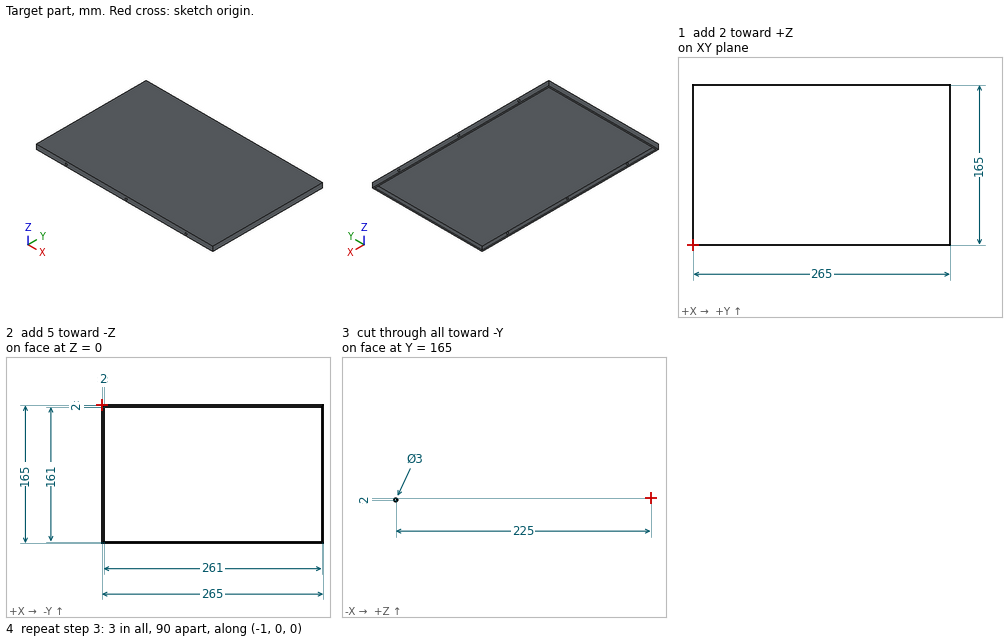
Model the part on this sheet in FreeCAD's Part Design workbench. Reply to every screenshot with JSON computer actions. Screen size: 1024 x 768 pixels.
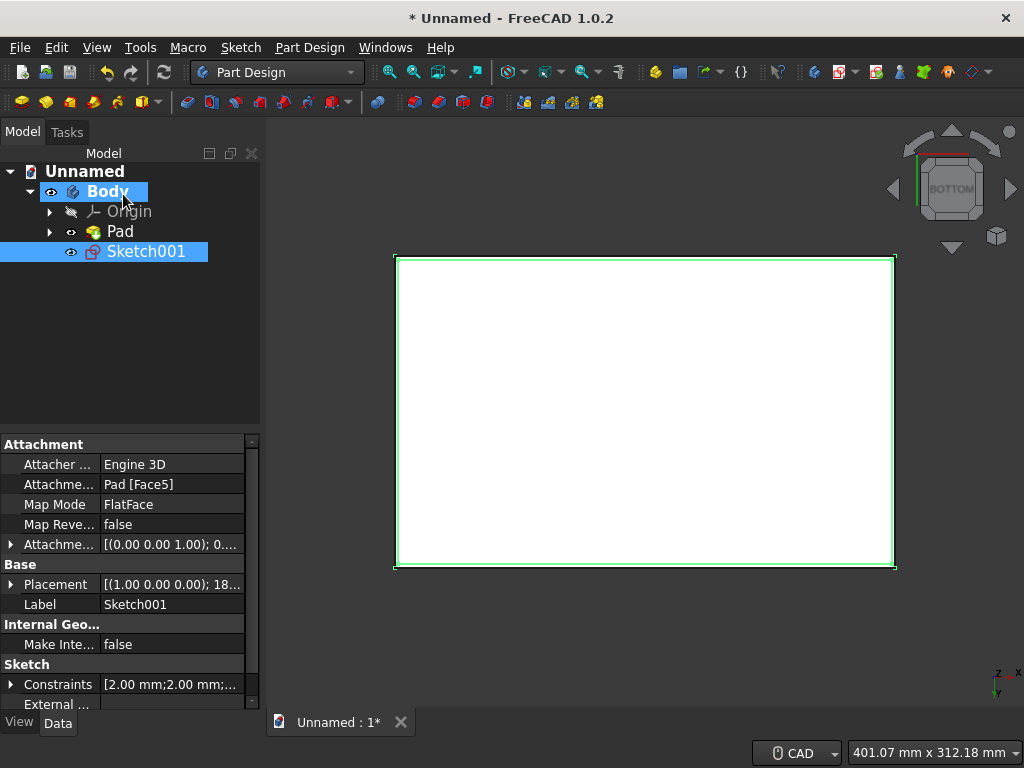
{"action": "left_click", "coordinate": [22, 102]}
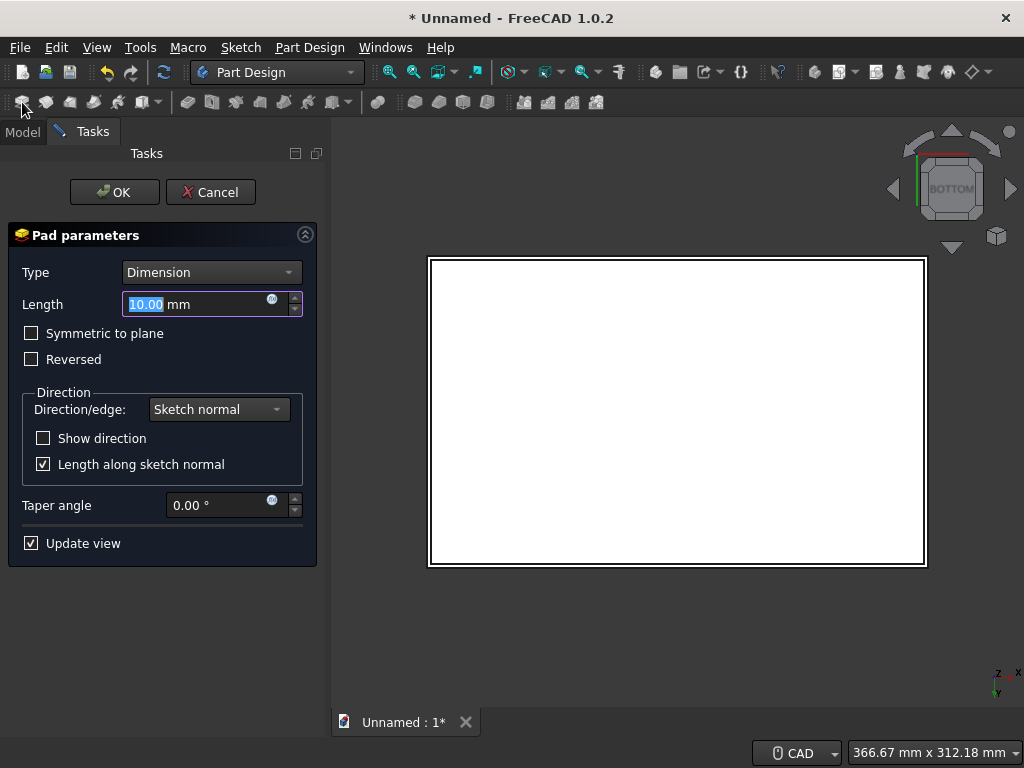
{"action": "type", "text": "5"}
{"action": "key", "text": "Tab"}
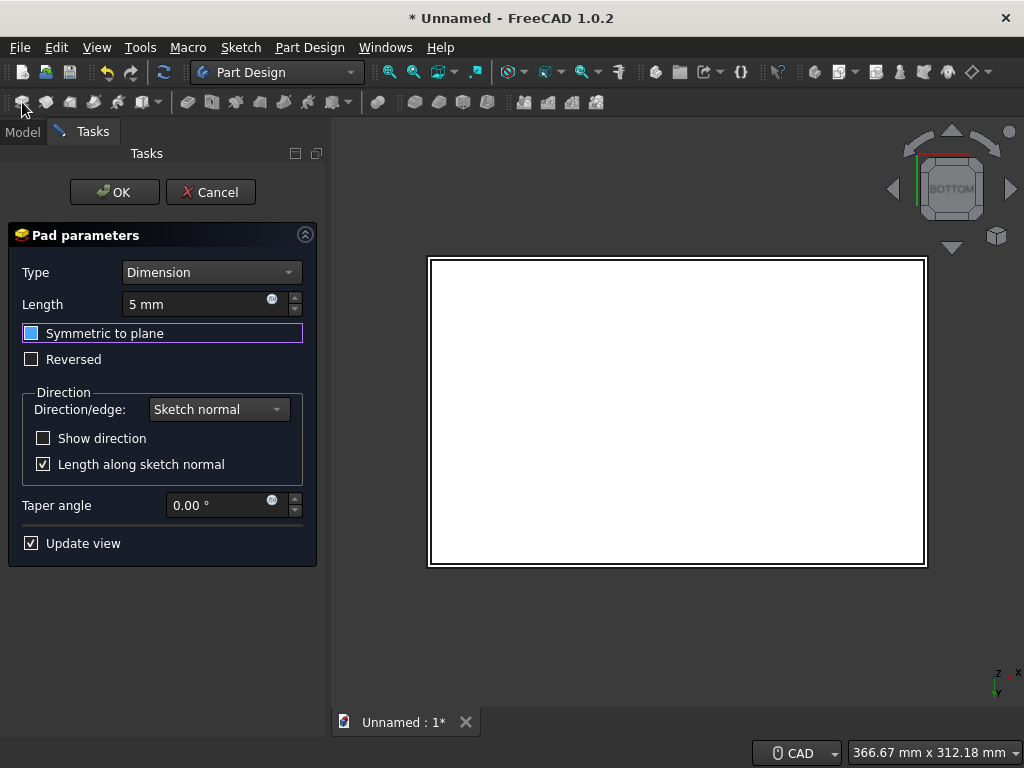
{"action": "left_click", "coordinate": [115, 192]}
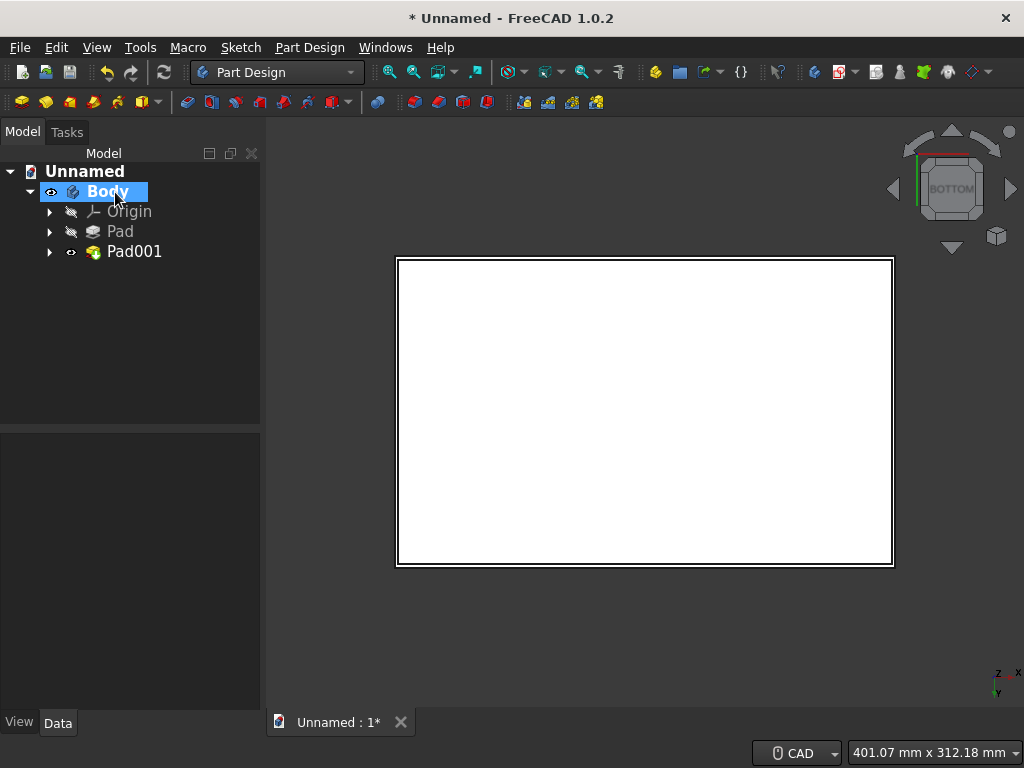
{"action": "key", "text": "4"}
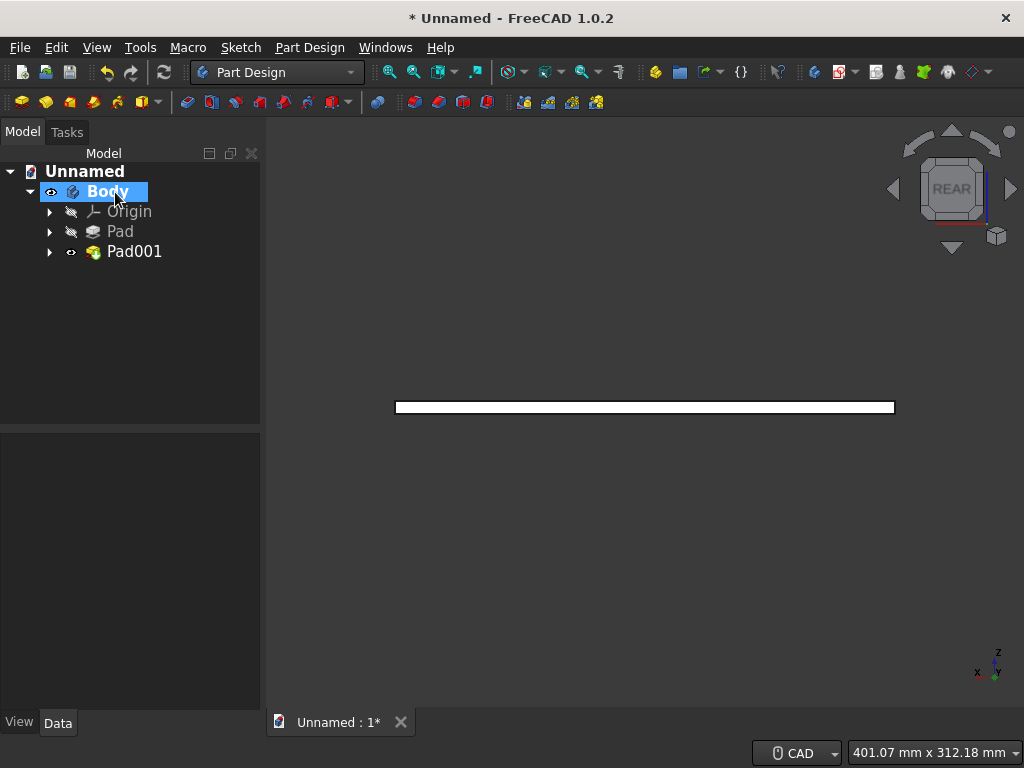
{"action": "scroll", "coordinate": [430, 406], "scroll_direction": "up", "scroll_amount": 3}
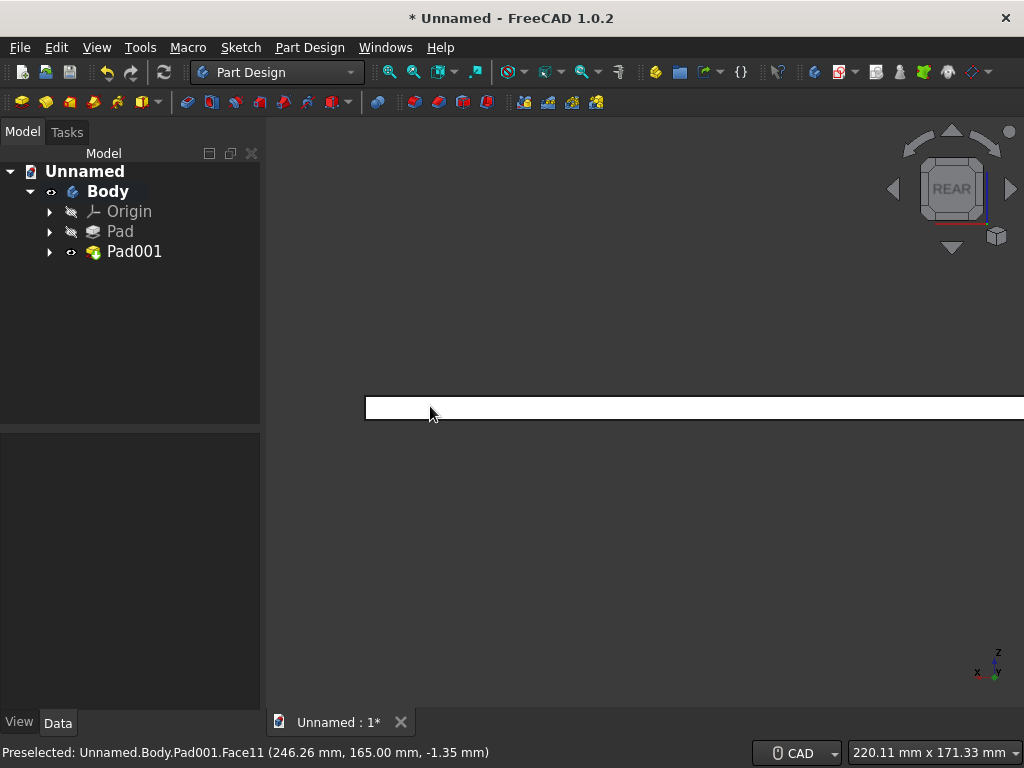
{"action": "left_click", "coordinate": [430, 407]}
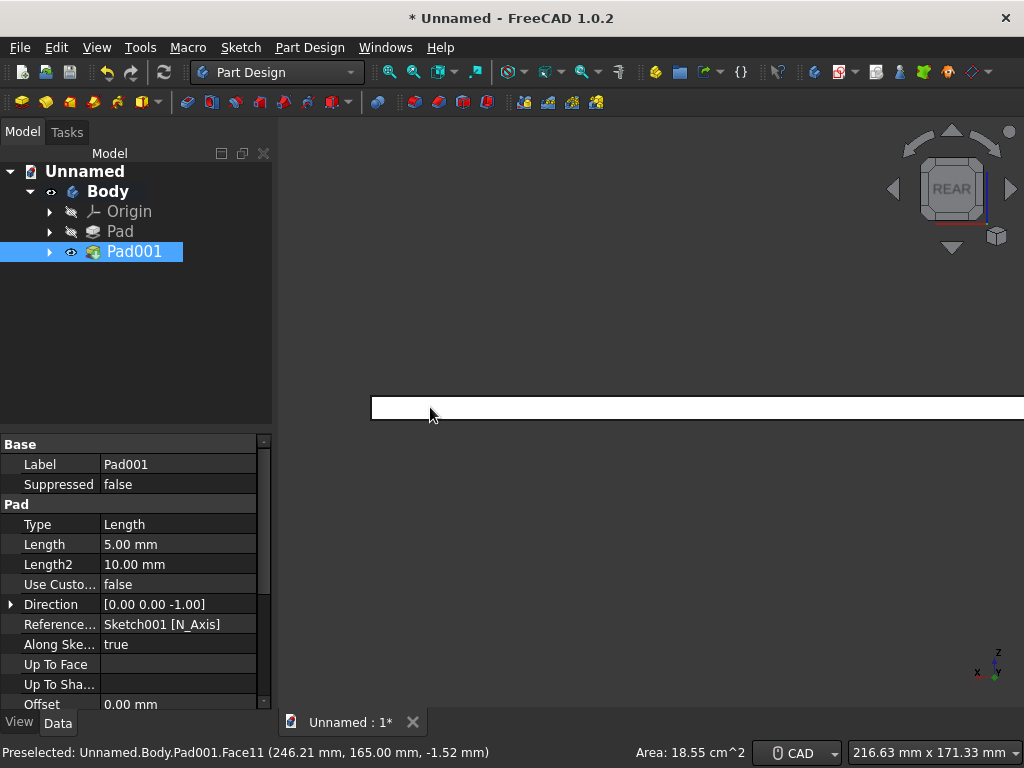
{"action": "left_click", "coordinate": [840, 72]}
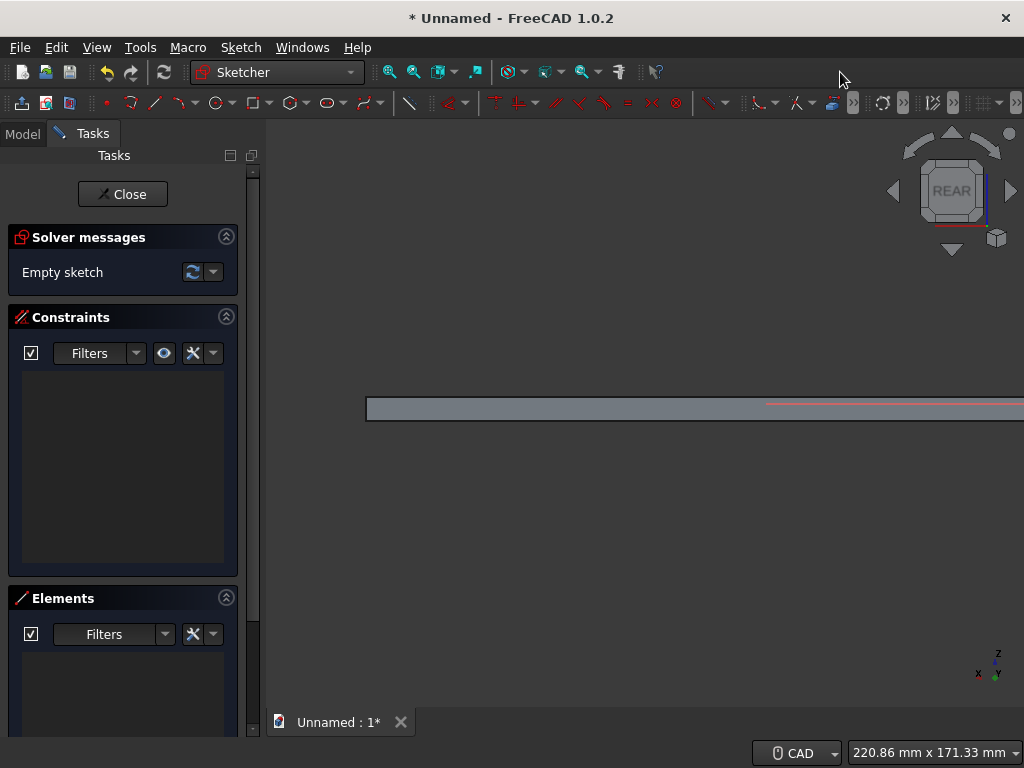
{"action": "scroll", "coordinate": [500, 411], "scroll_direction": "up", "scroll_amount": 15}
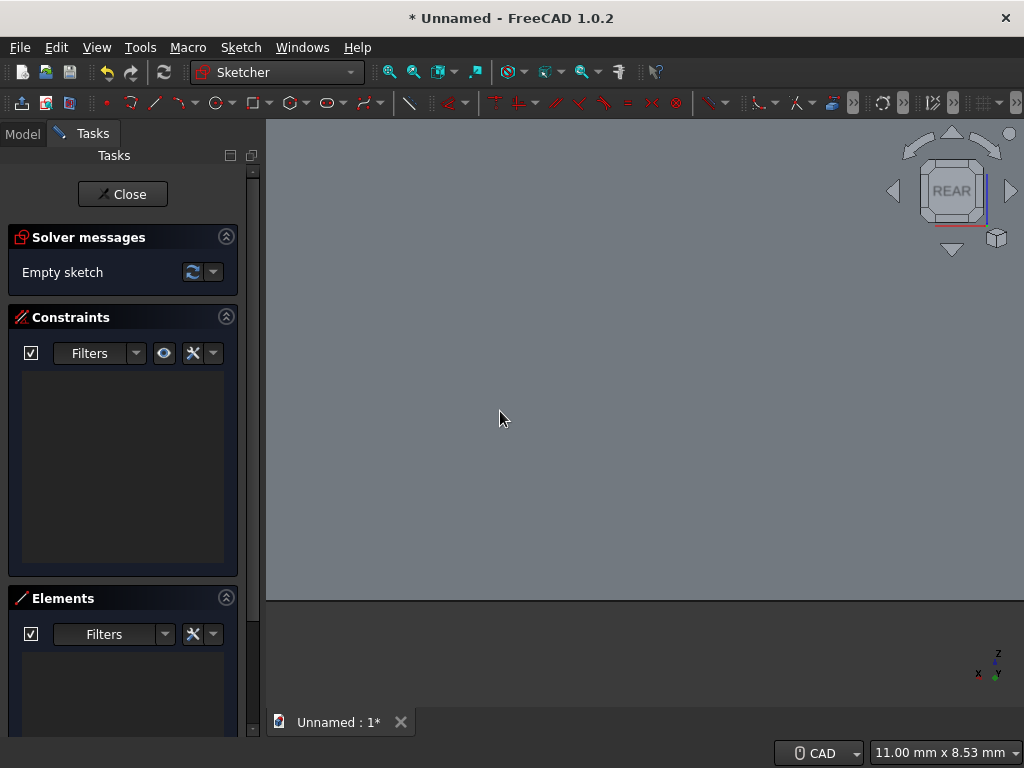
{"action": "scroll", "coordinate": [550, 372], "scroll_direction": "up", "scroll_amount": 3}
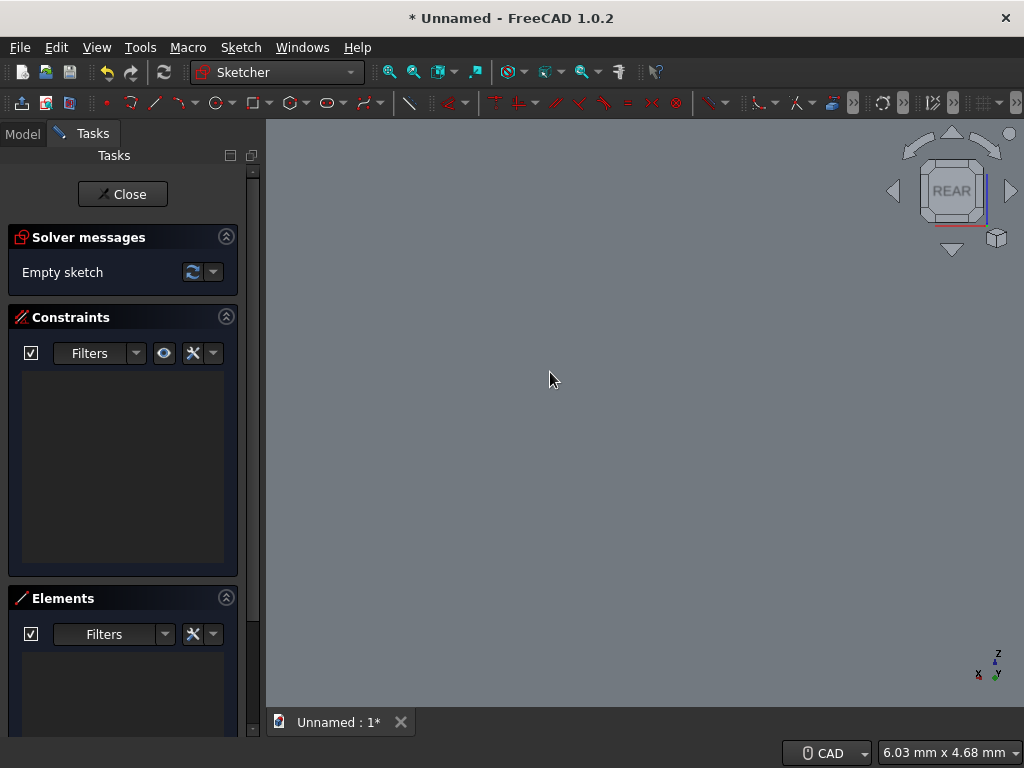
{"action": "key", "text": "g c"}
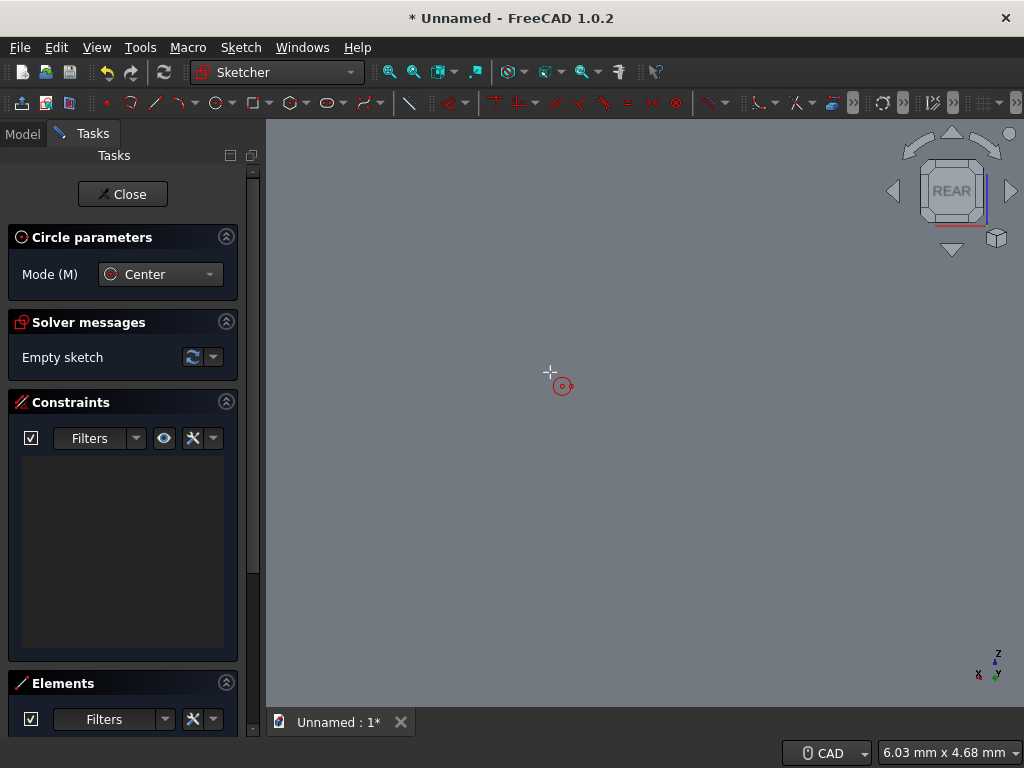
{"action": "left_click", "coordinate": [576, 413]}
{"action": "left_click", "coordinate": [710, 279]}
{"action": "key", "text": "Escape"}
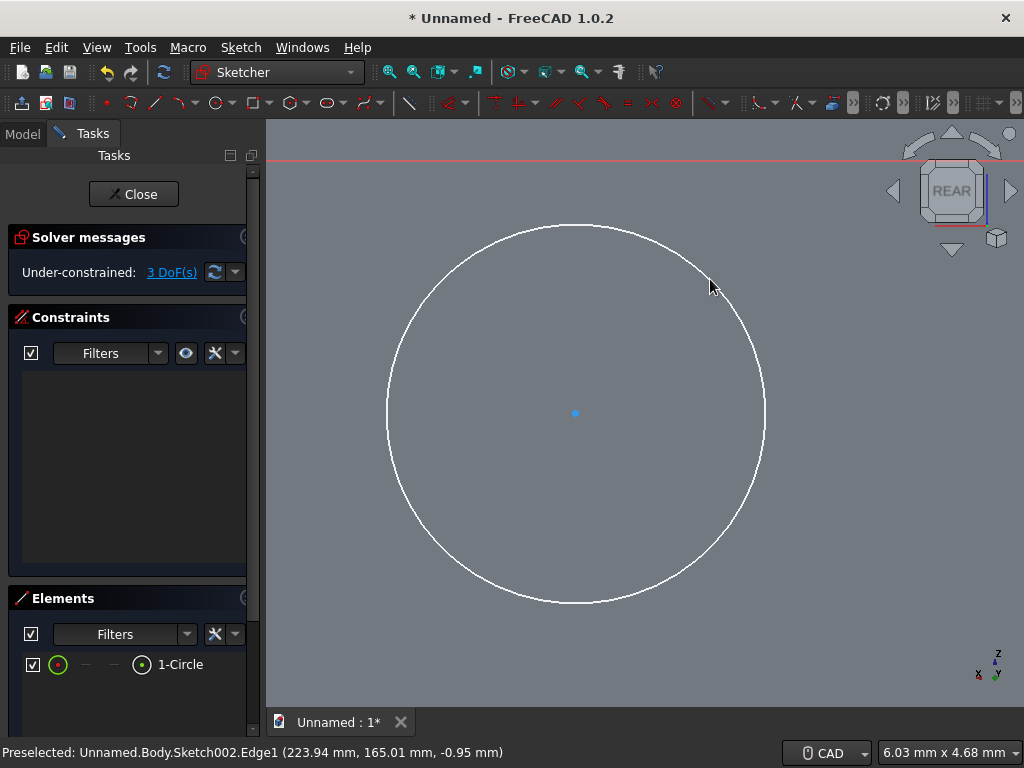
{"action": "key", "text": "d"}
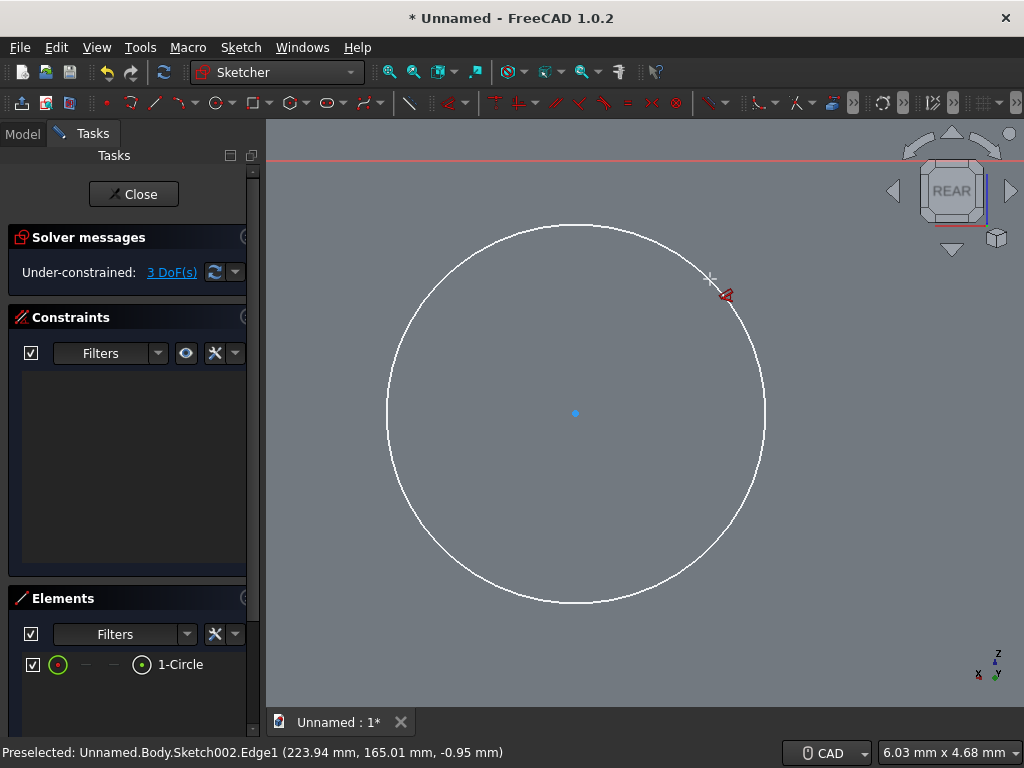
{"action": "left_click", "coordinate": [710, 280]}
{"action": "left_click", "coordinate": [733, 257]}